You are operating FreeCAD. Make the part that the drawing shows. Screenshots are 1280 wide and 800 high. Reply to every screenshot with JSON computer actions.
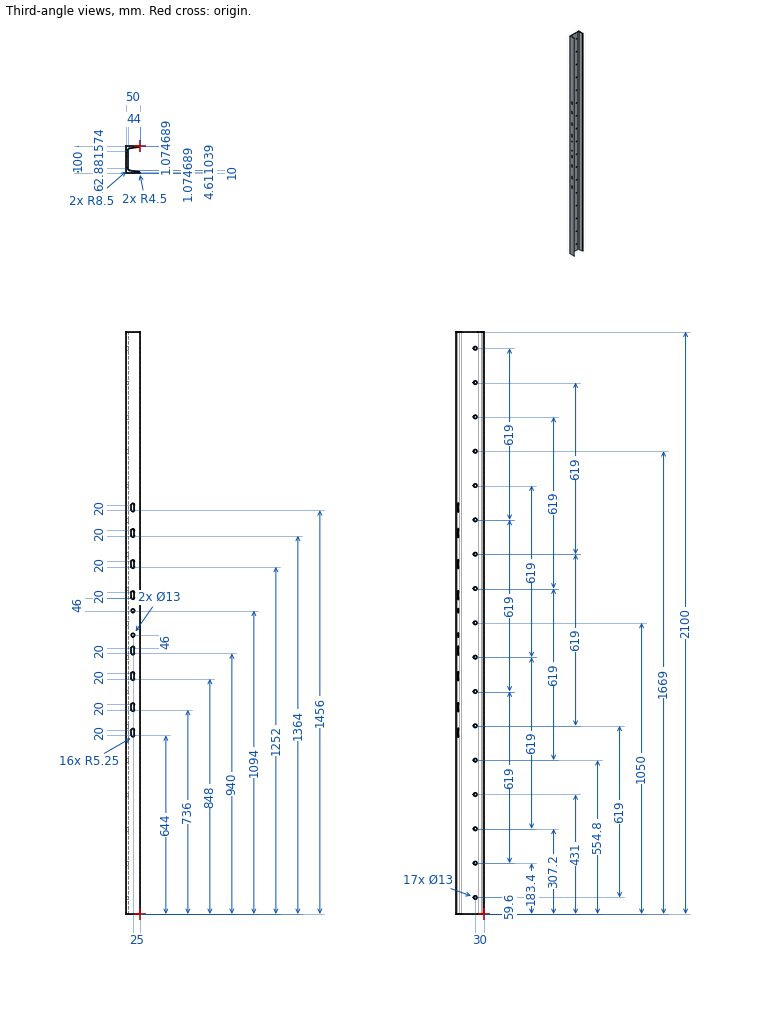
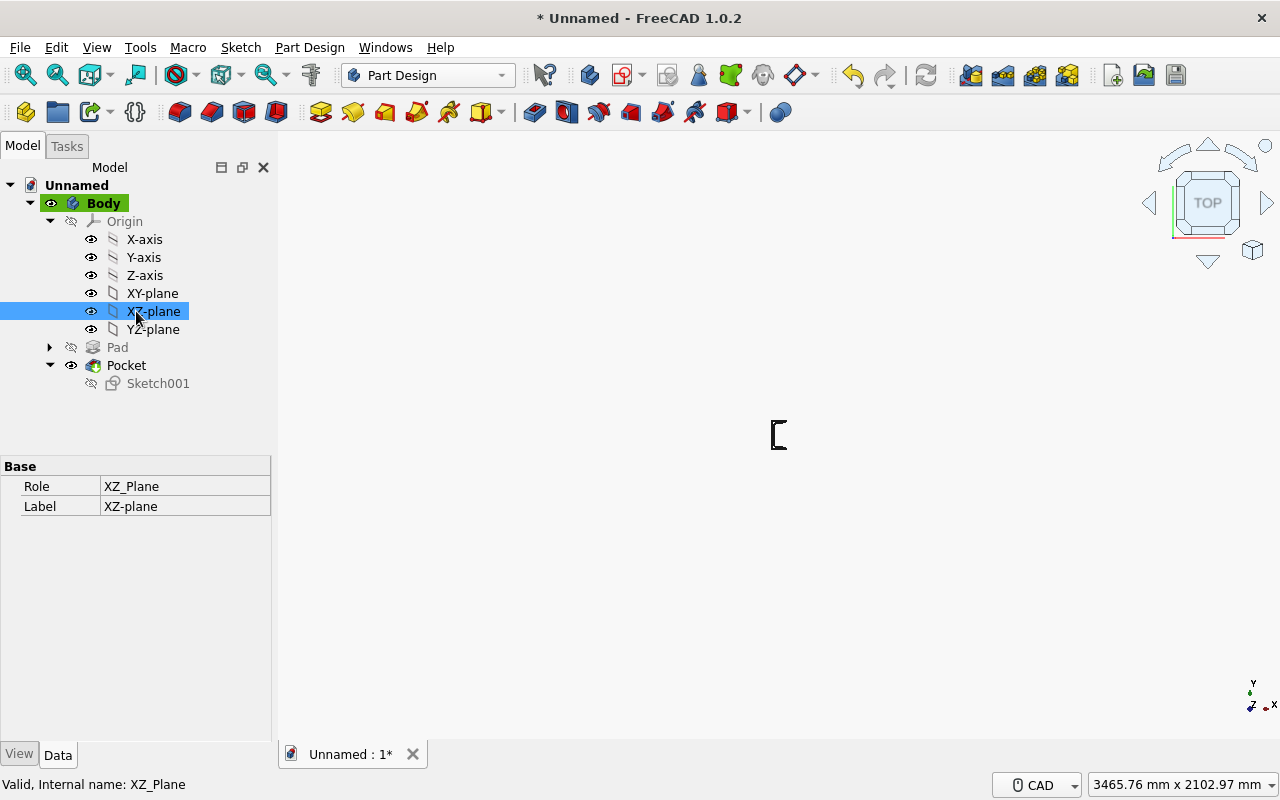
{"action": "left_click", "coordinate": [796, 76]}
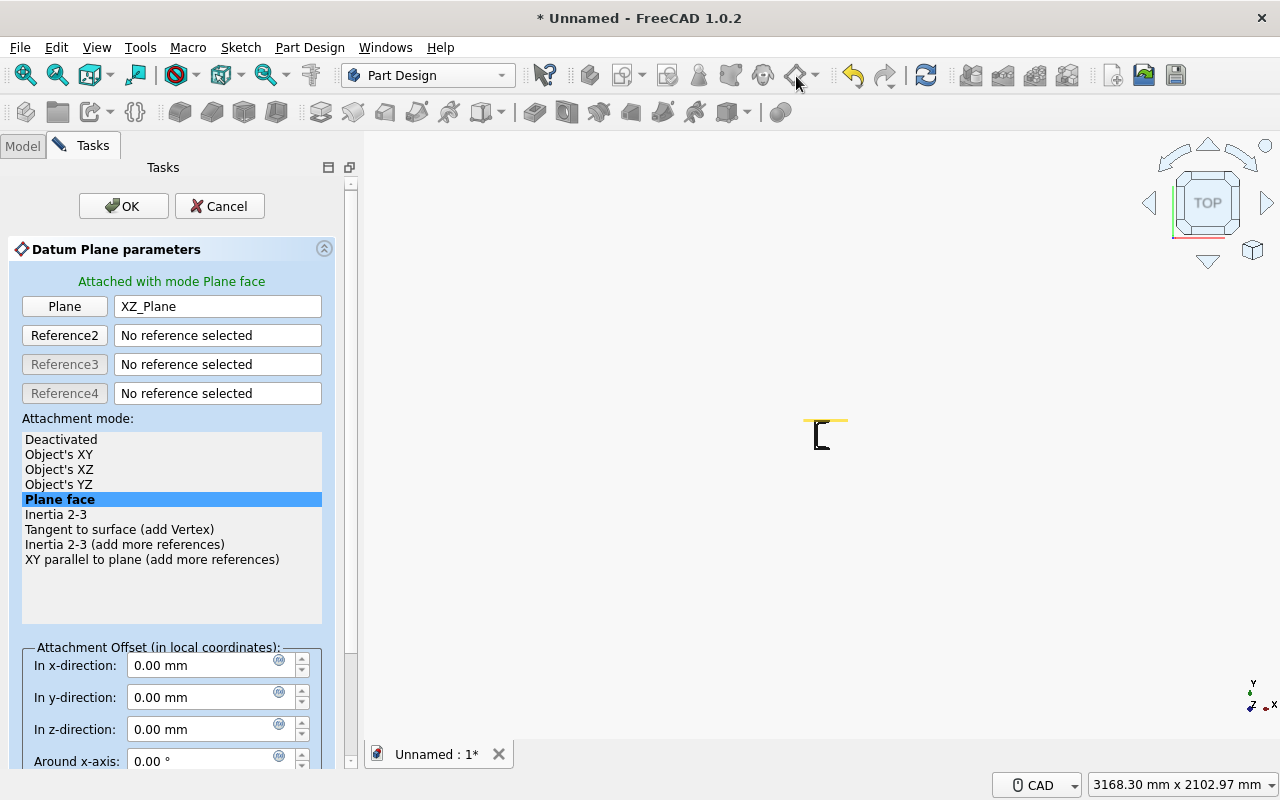
{"action": "triple_click", "coordinate": [210, 729]}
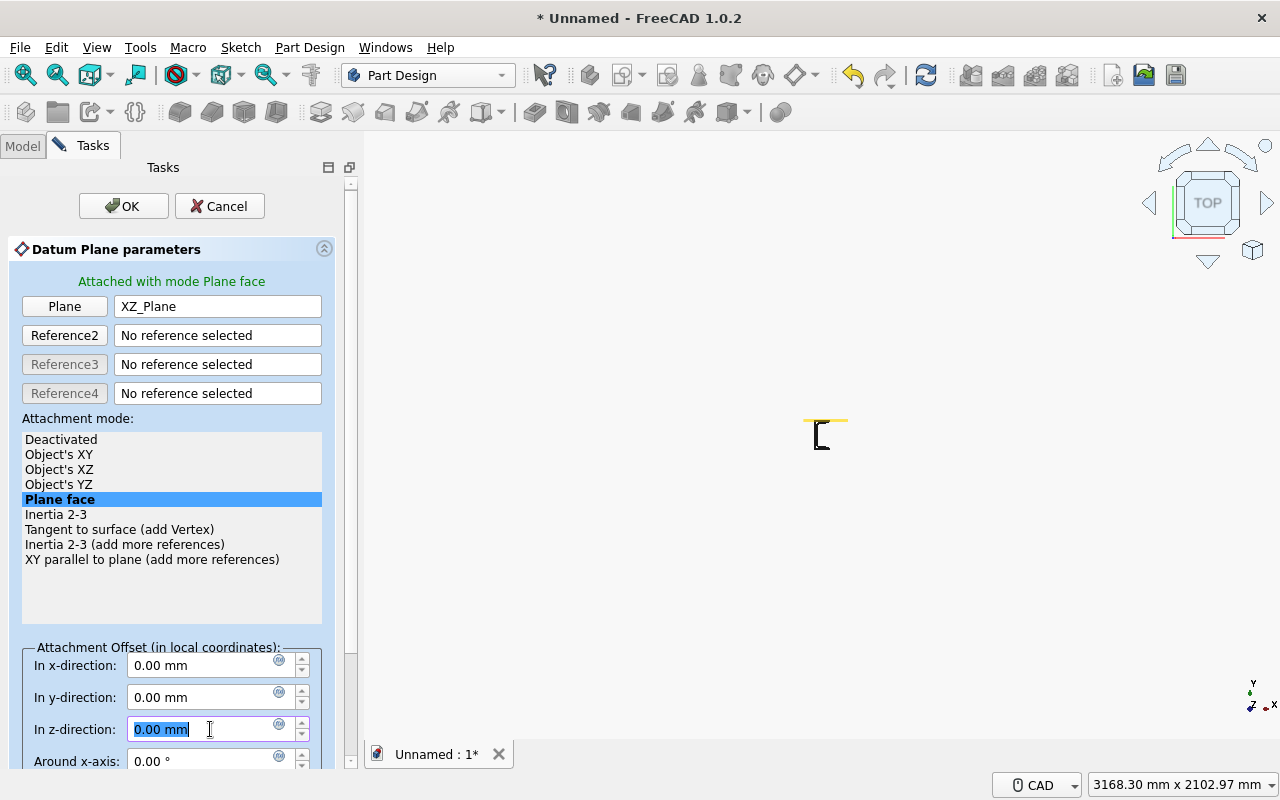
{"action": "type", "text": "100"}
{"action": "key", "text": "Tab"}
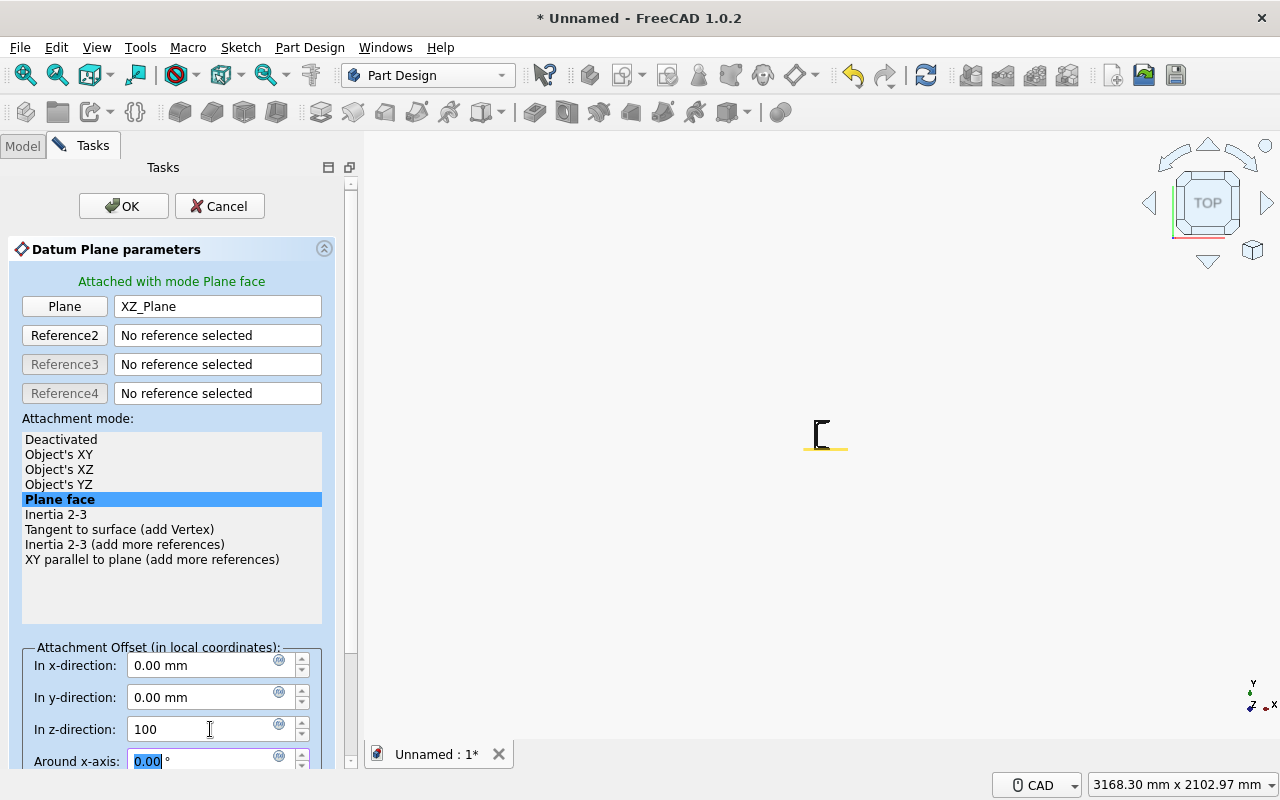
{"action": "left_click", "coordinate": [124, 206]}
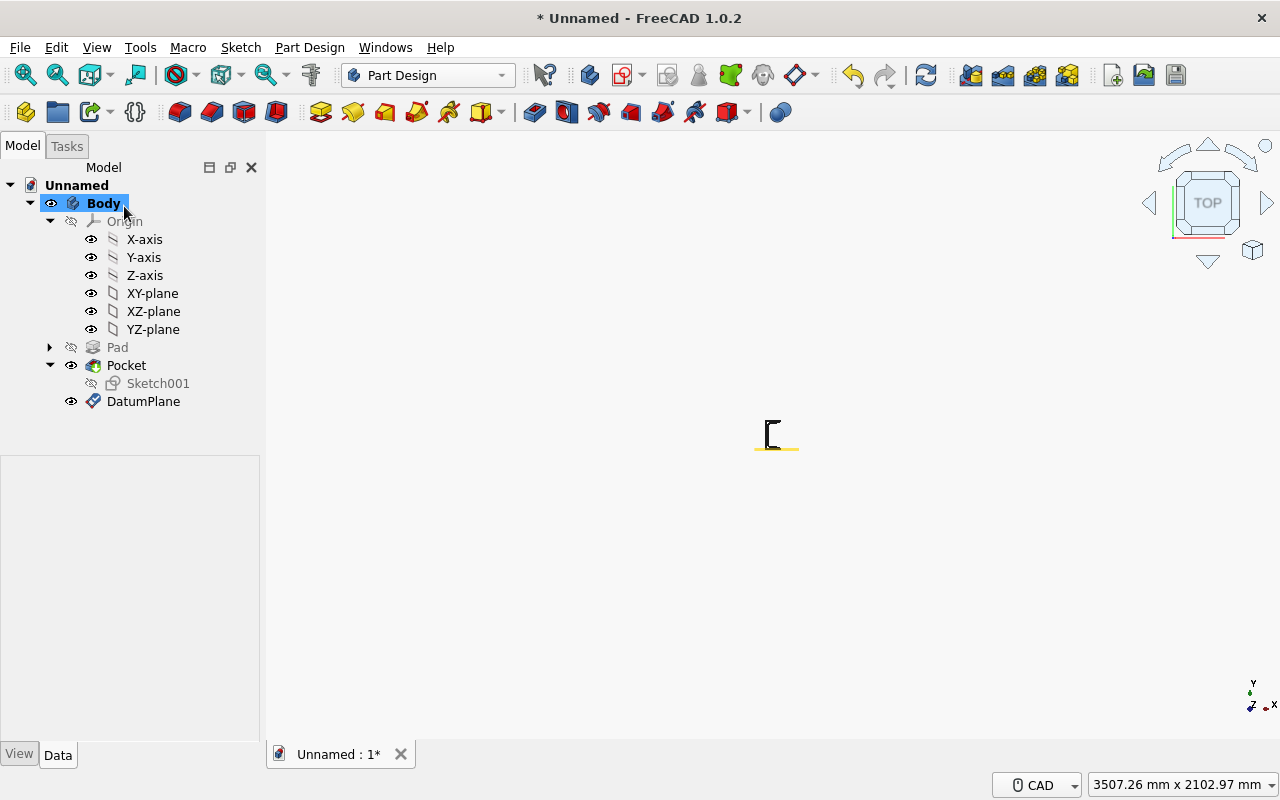
{"action": "left_click", "coordinate": [116, 401]}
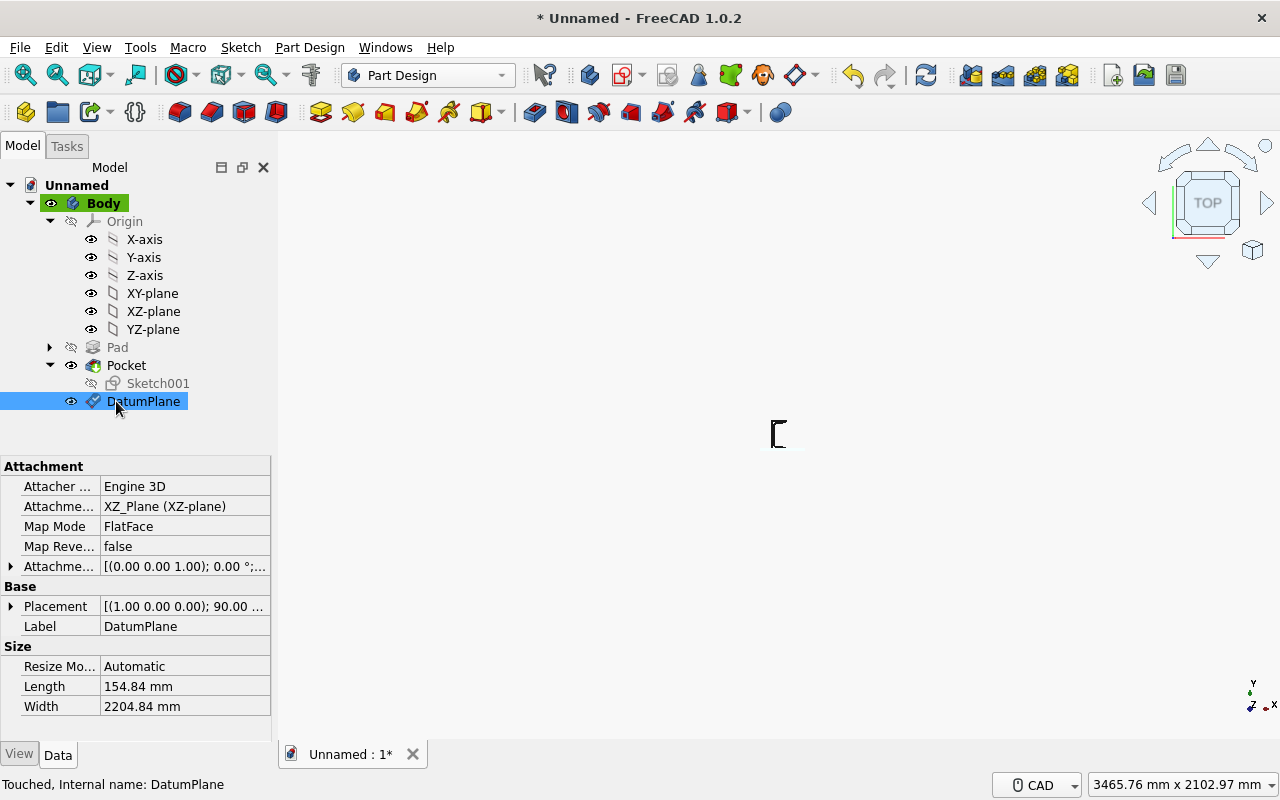
{"action": "left_click", "coordinate": [622, 76]}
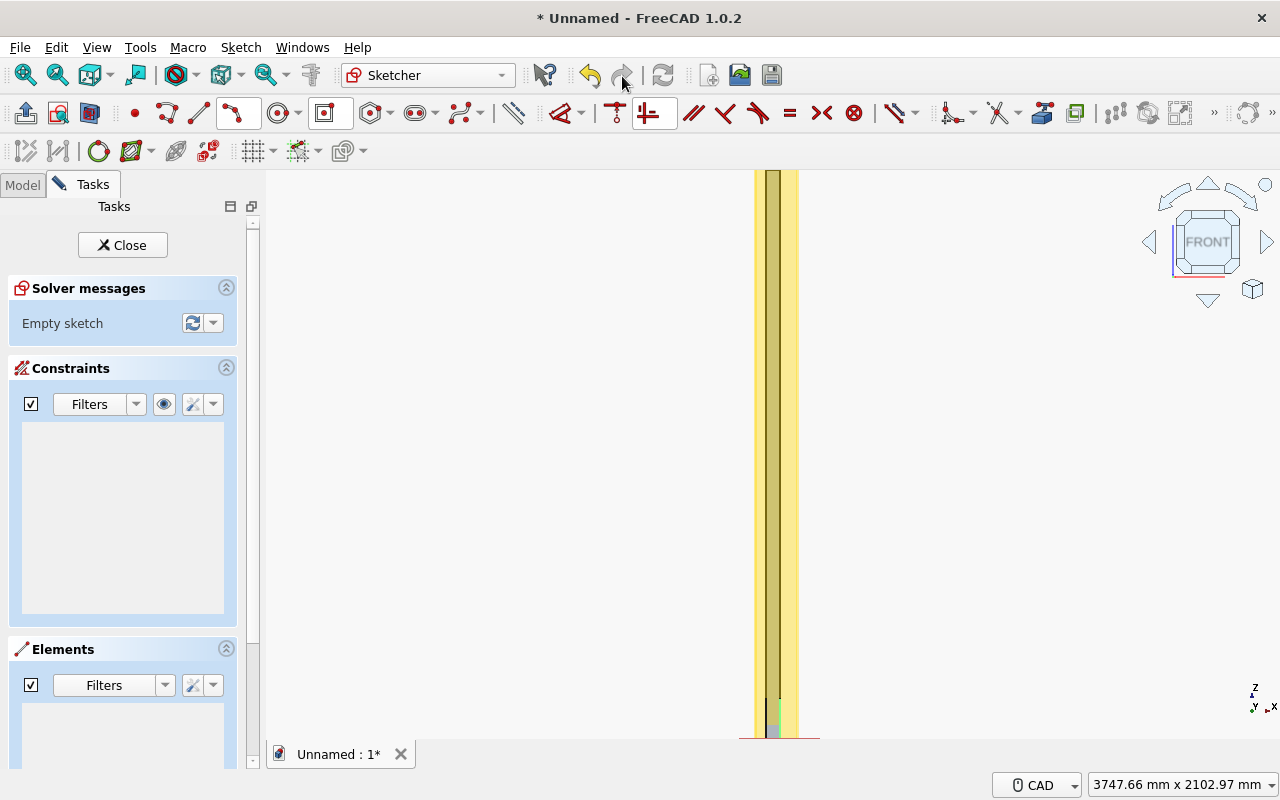
{"action": "scroll", "coordinate": [384, 198], "scroll_direction": "down", "scroll_amount": 1}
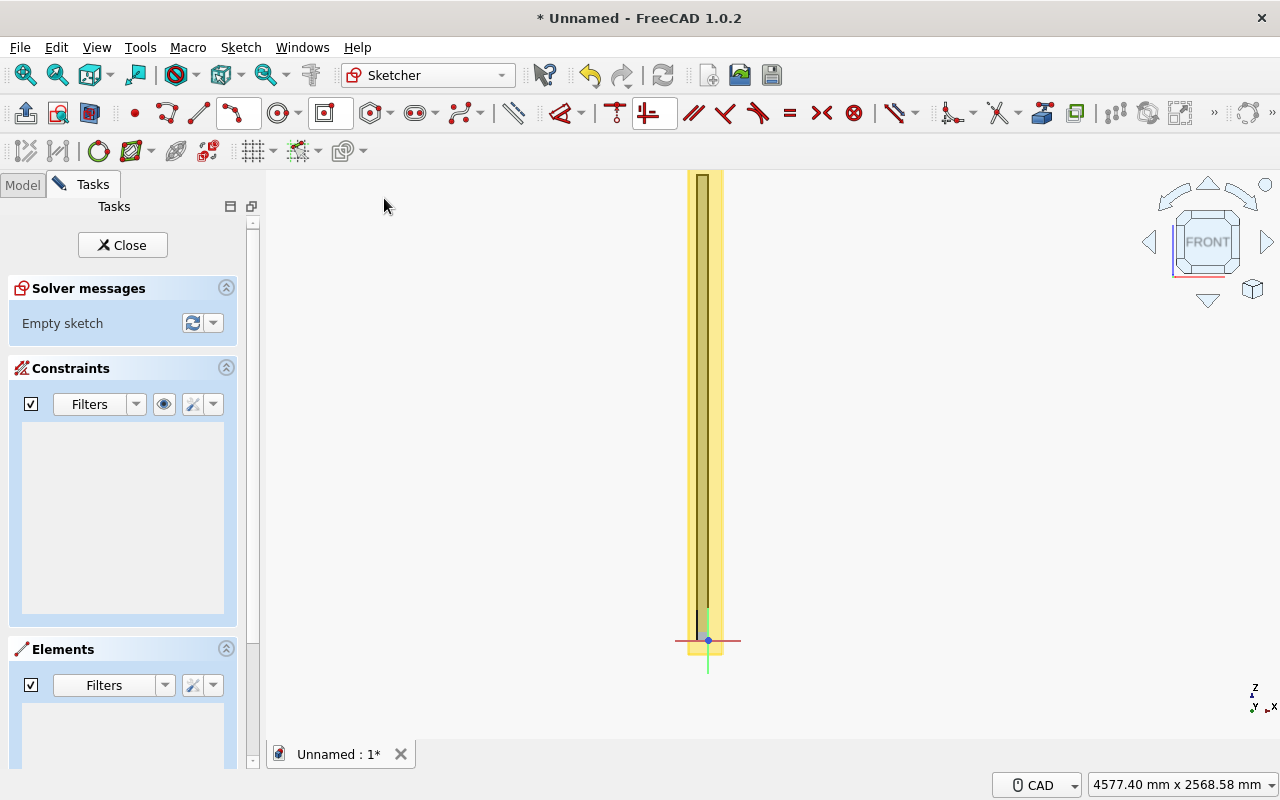
{"action": "left_click", "coordinate": [416, 114]}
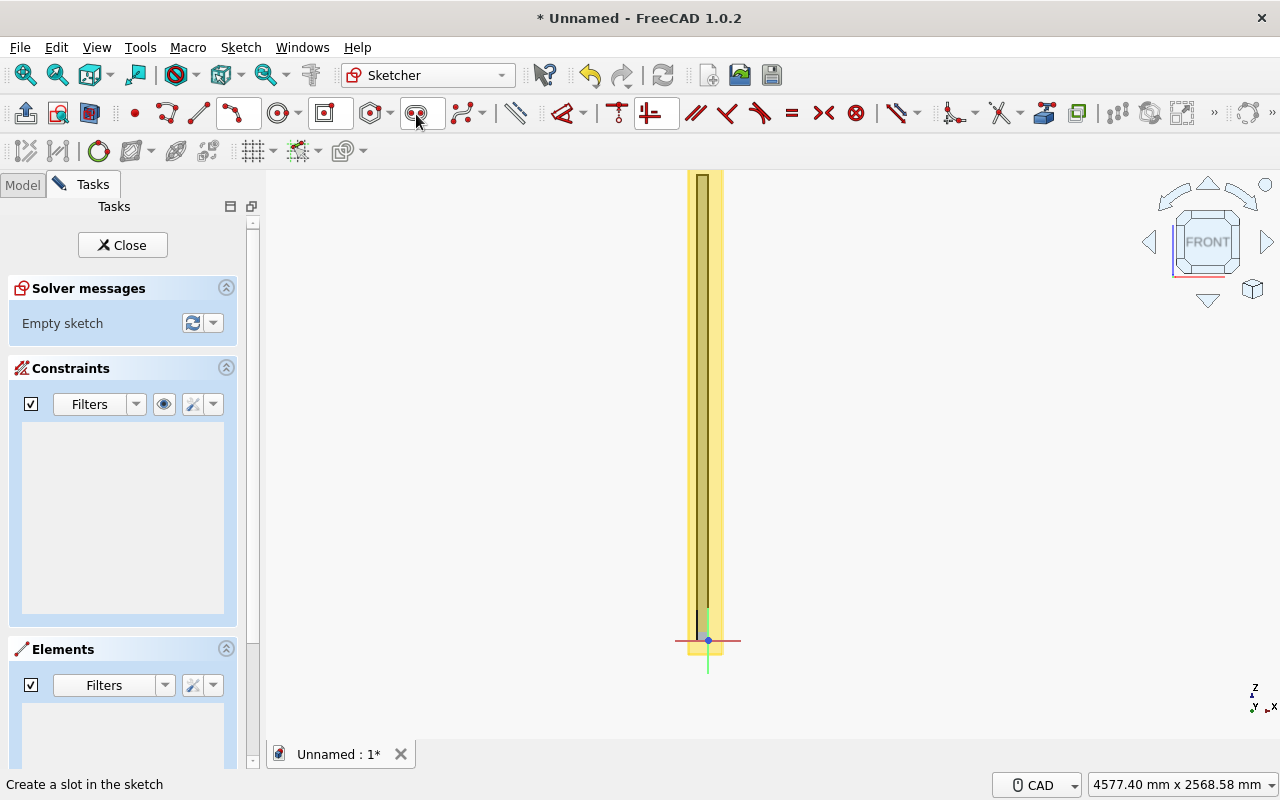
{"action": "scroll", "coordinate": [703, 498], "scroll_direction": "up", "scroll_amount": 15}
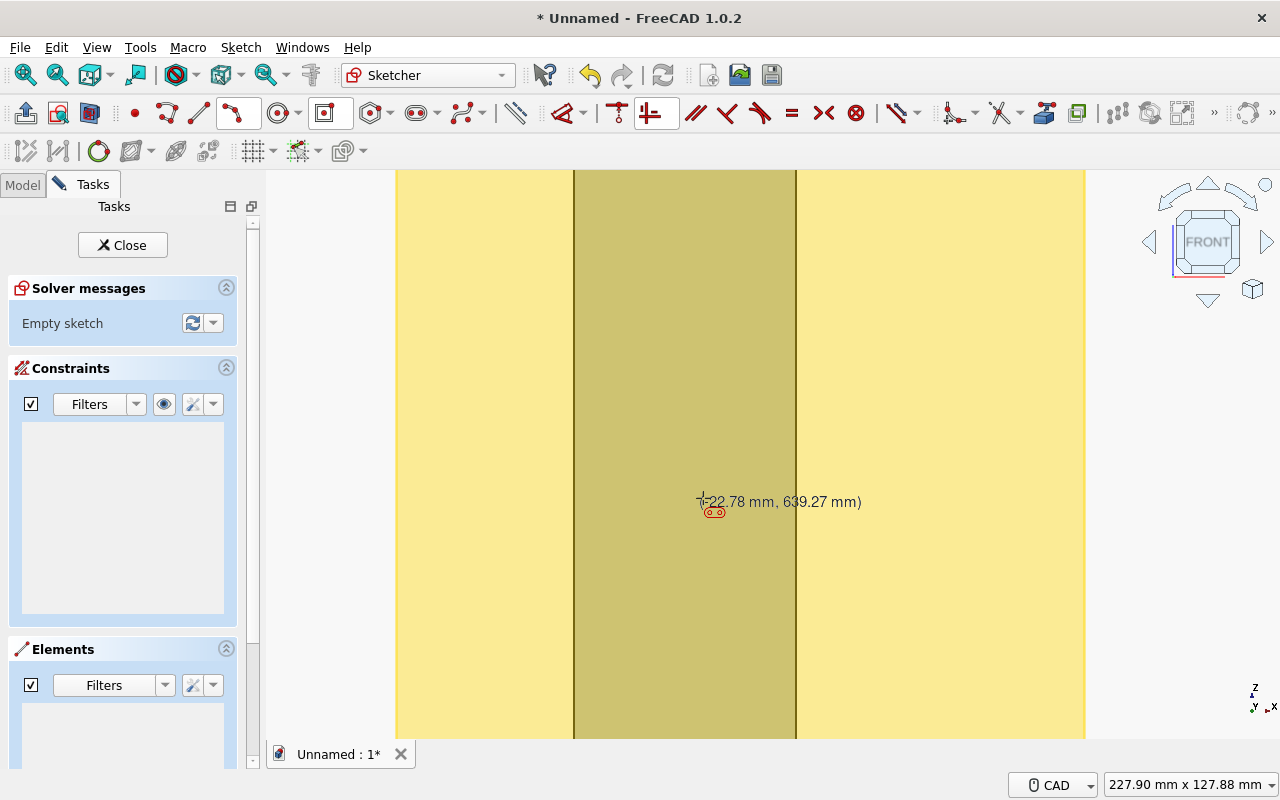
{"action": "scroll", "coordinate": [703, 475], "scroll_direction": "down", "scroll_amount": 15}